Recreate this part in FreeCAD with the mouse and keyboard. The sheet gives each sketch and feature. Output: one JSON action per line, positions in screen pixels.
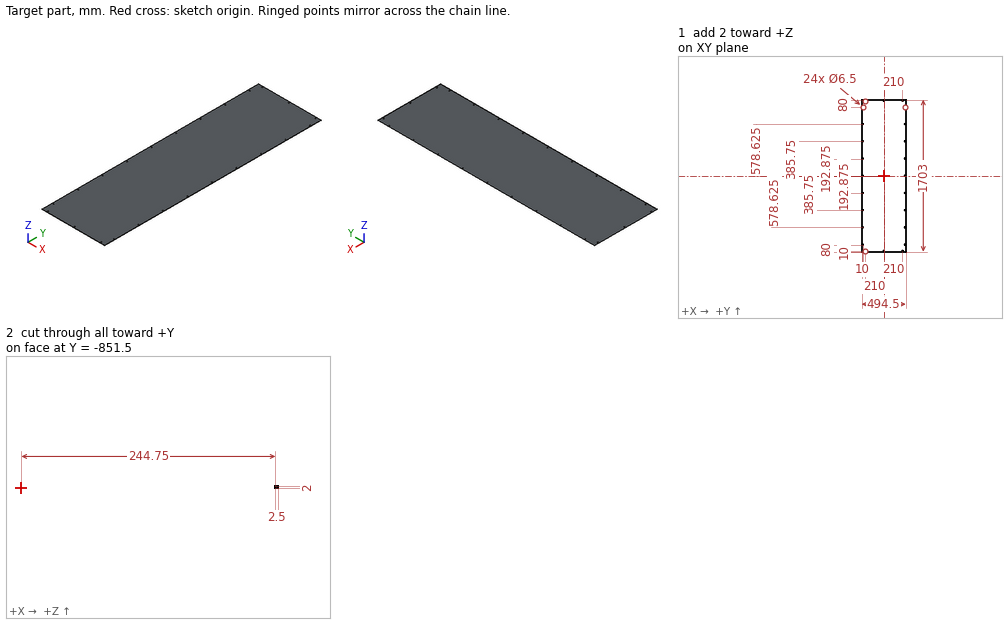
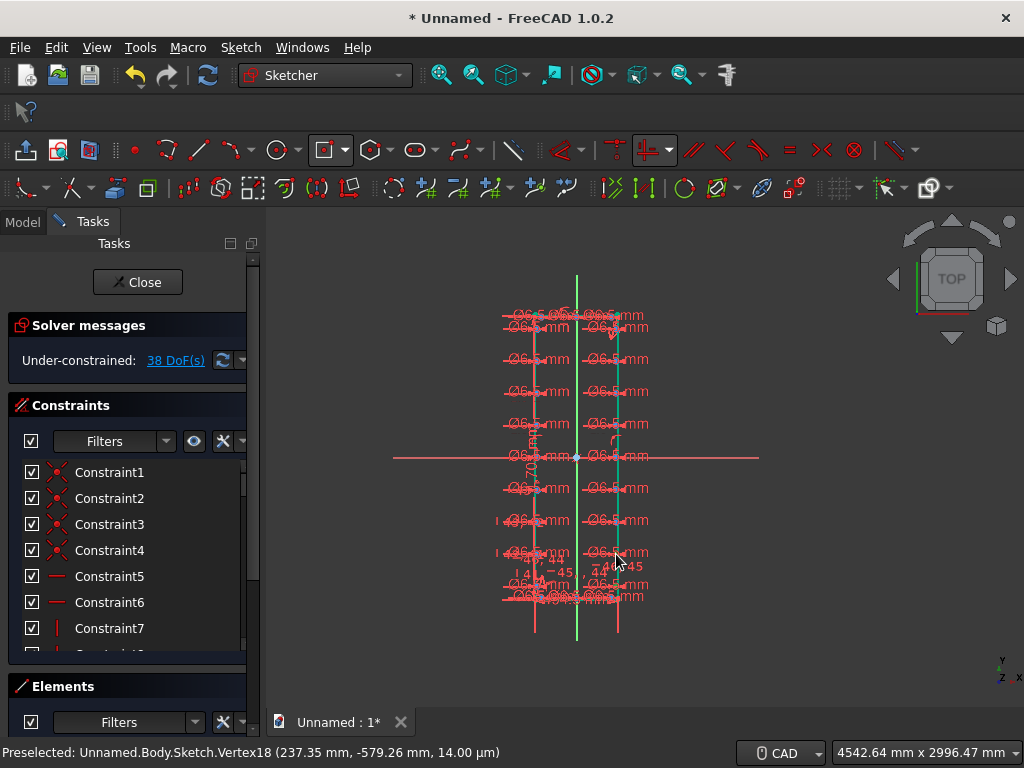
{"action": "key", "text": "v"}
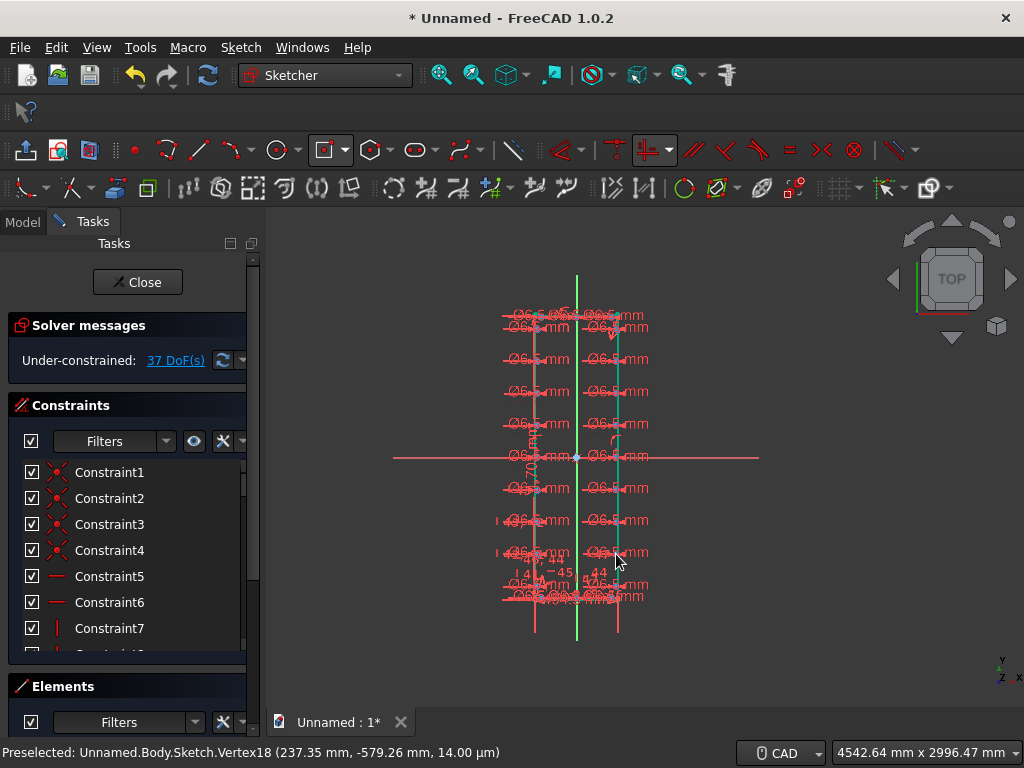
{"action": "left_click", "coordinate": [537, 554]}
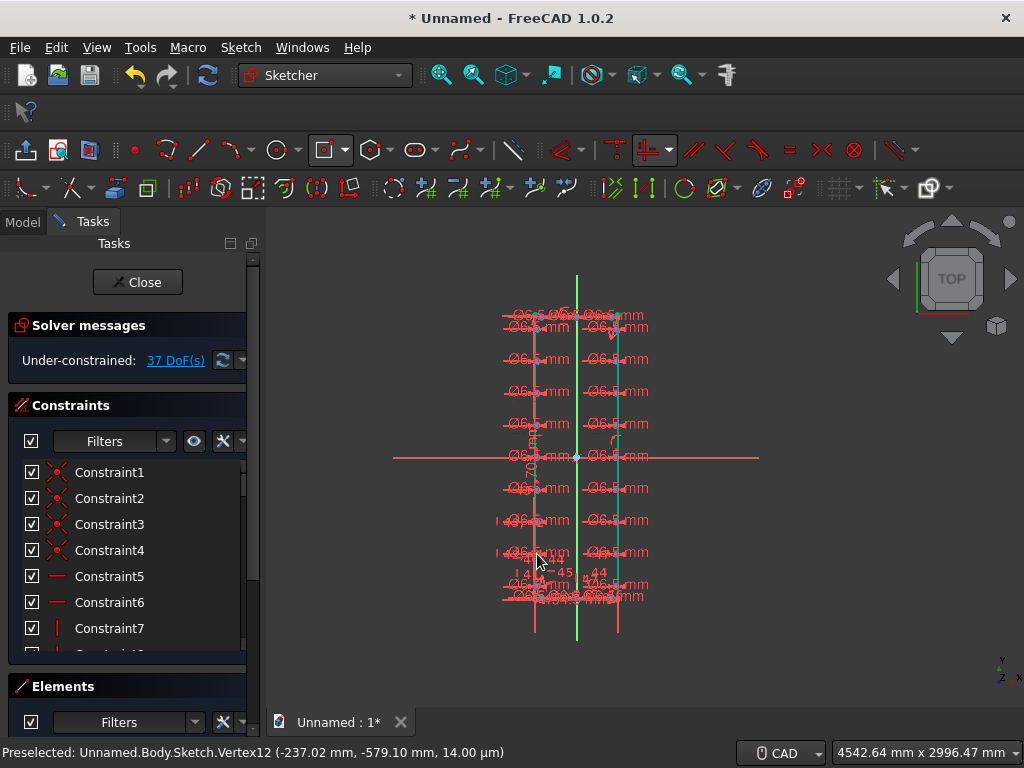
{"action": "left_click", "coordinate": [616, 554]}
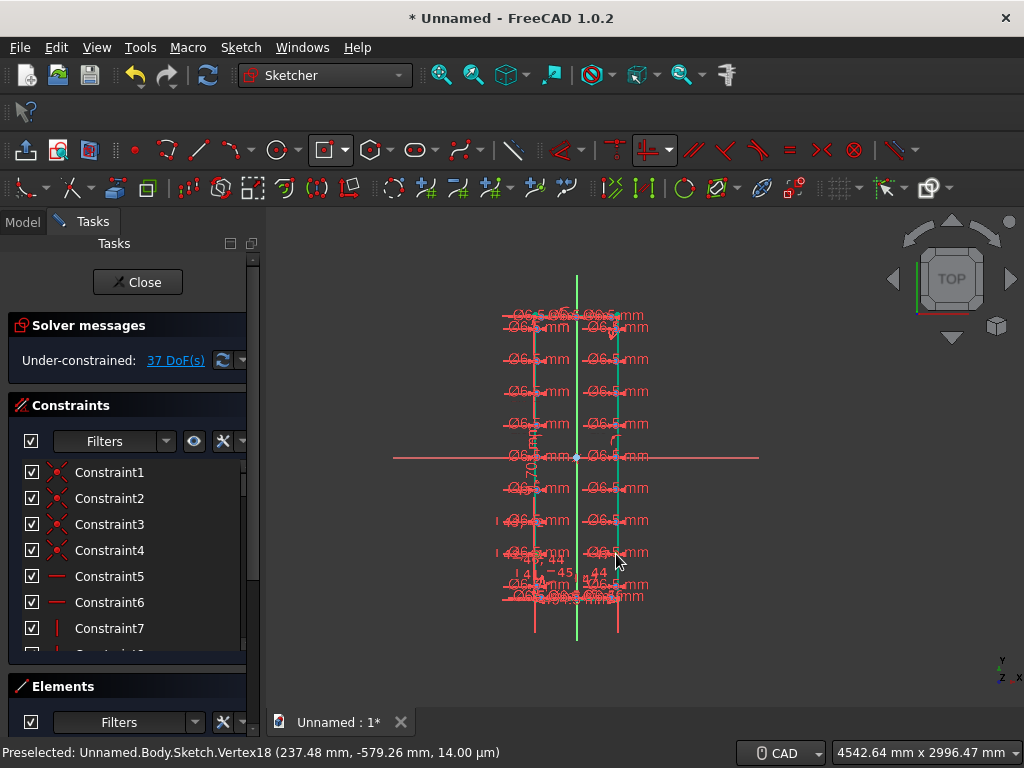
{"action": "key", "text": "h"}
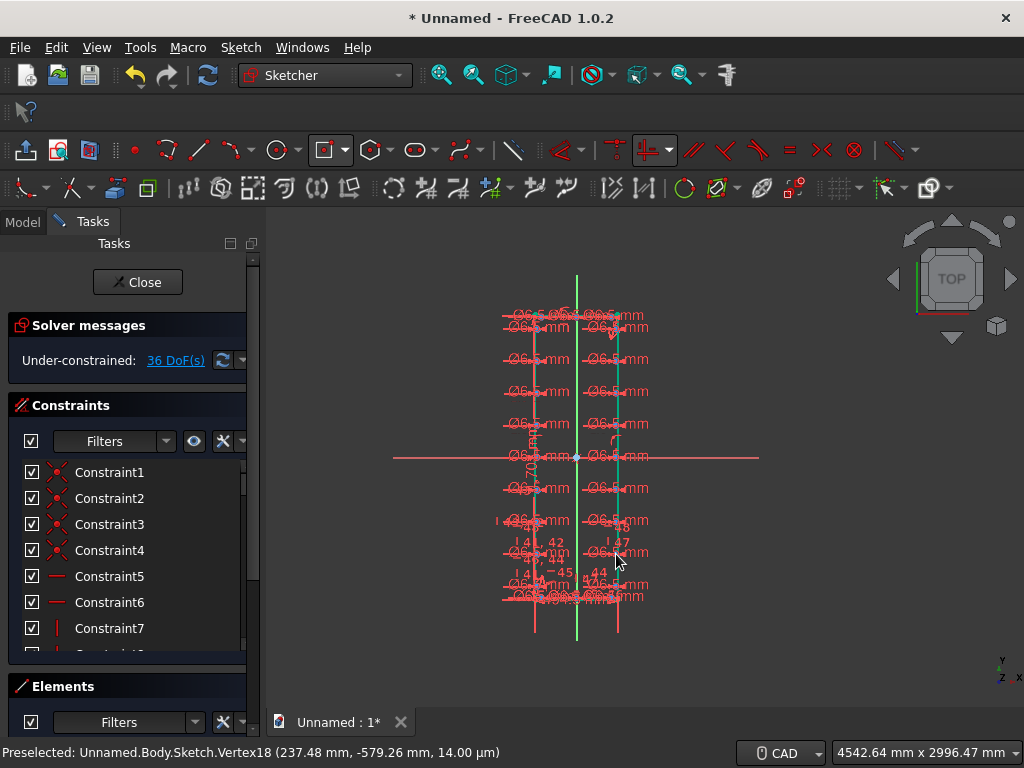
{"action": "left_click", "coordinate": [616, 554]}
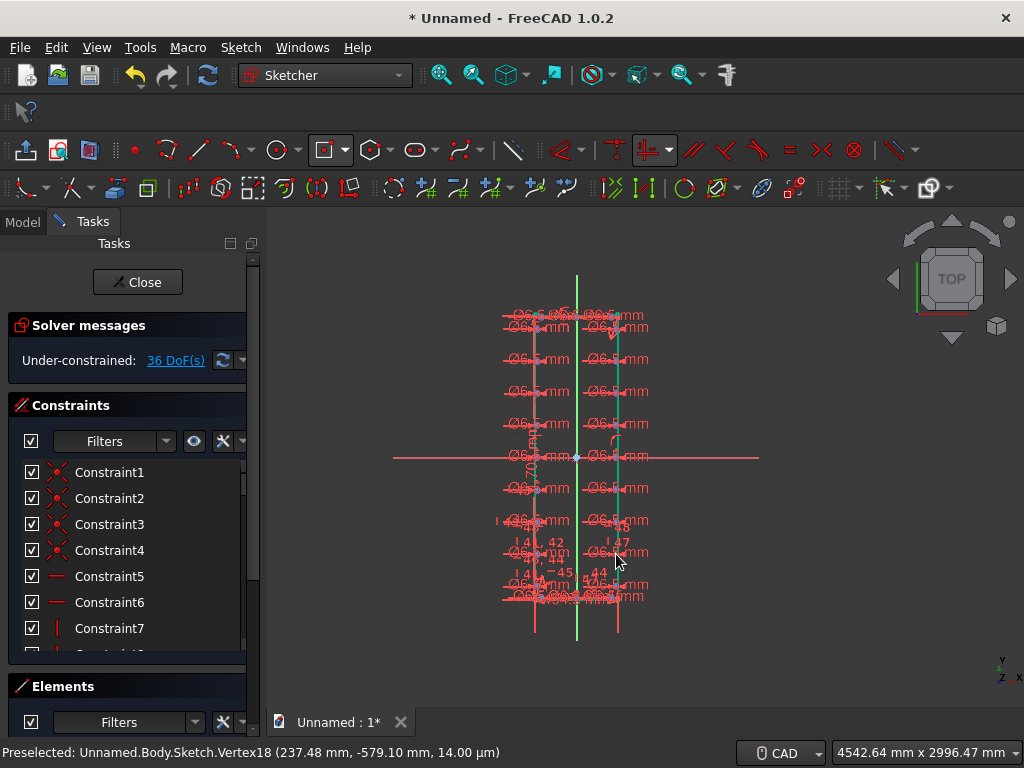
{"action": "scroll", "coordinate": [616, 522], "scroll_direction": "up", "scroll_amount": 4}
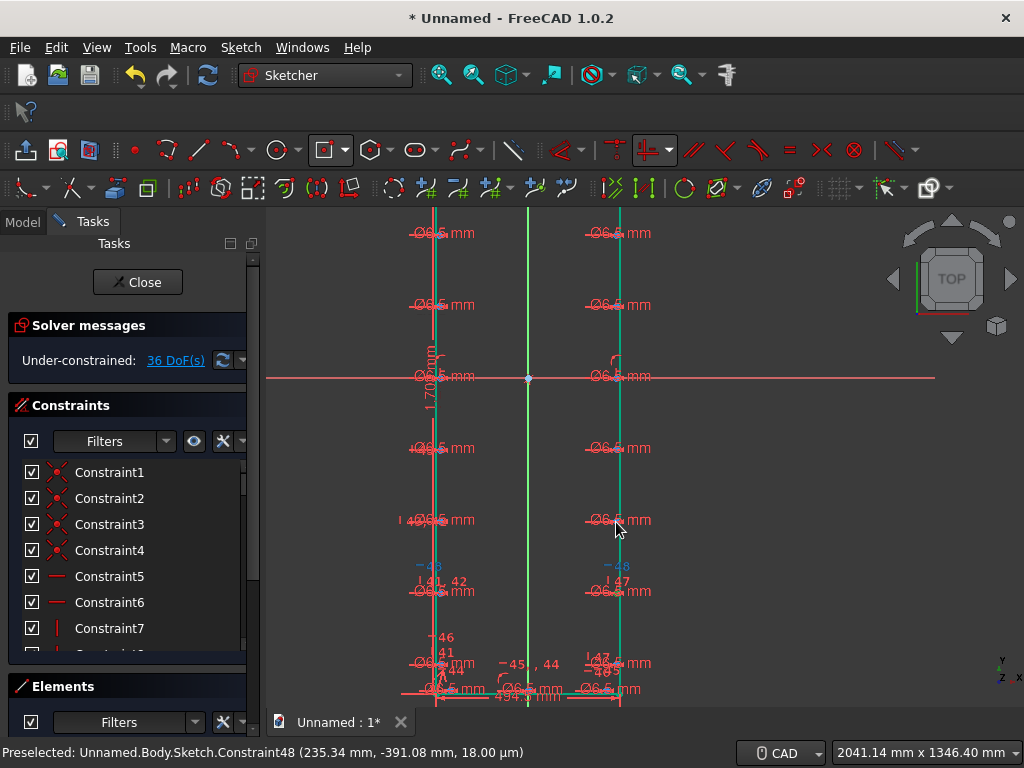
{"action": "left_click", "coordinate": [616, 522]}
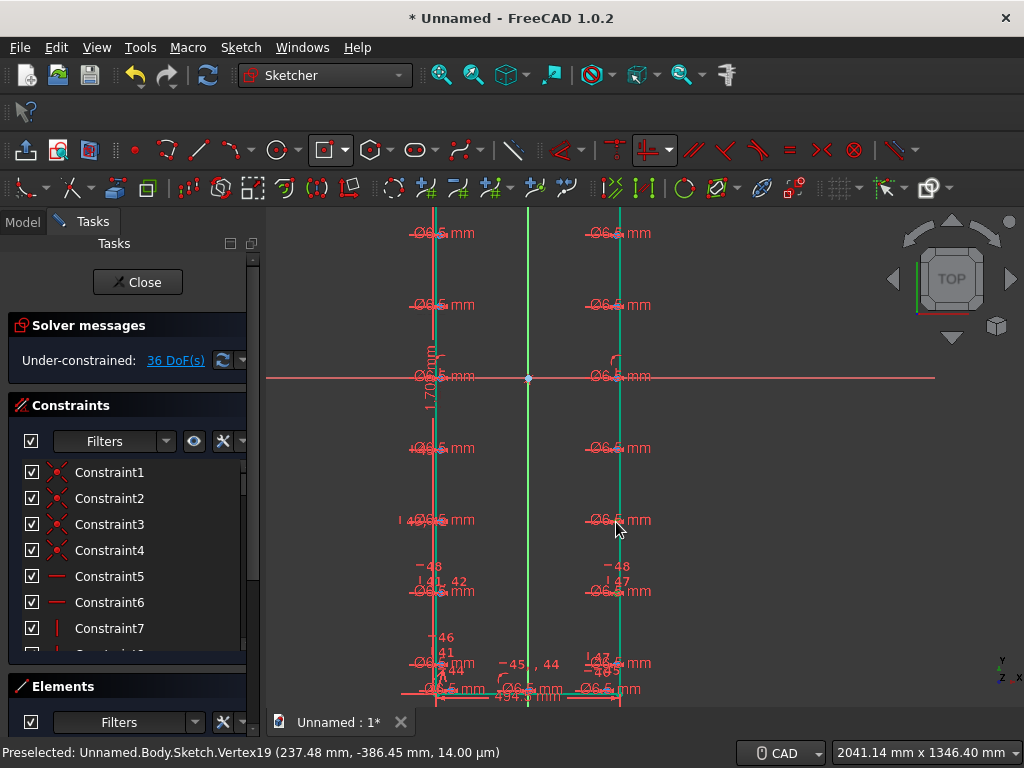
{"action": "key", "text": "v"}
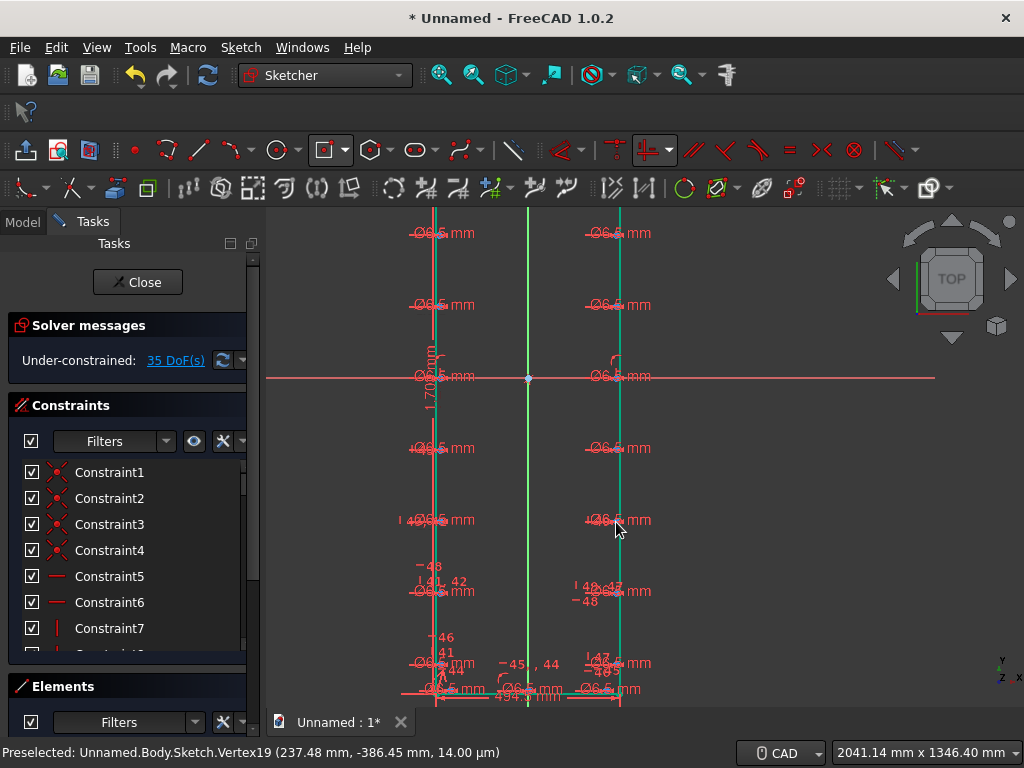
{"action": "left_click", "coordinate": [440, 522]}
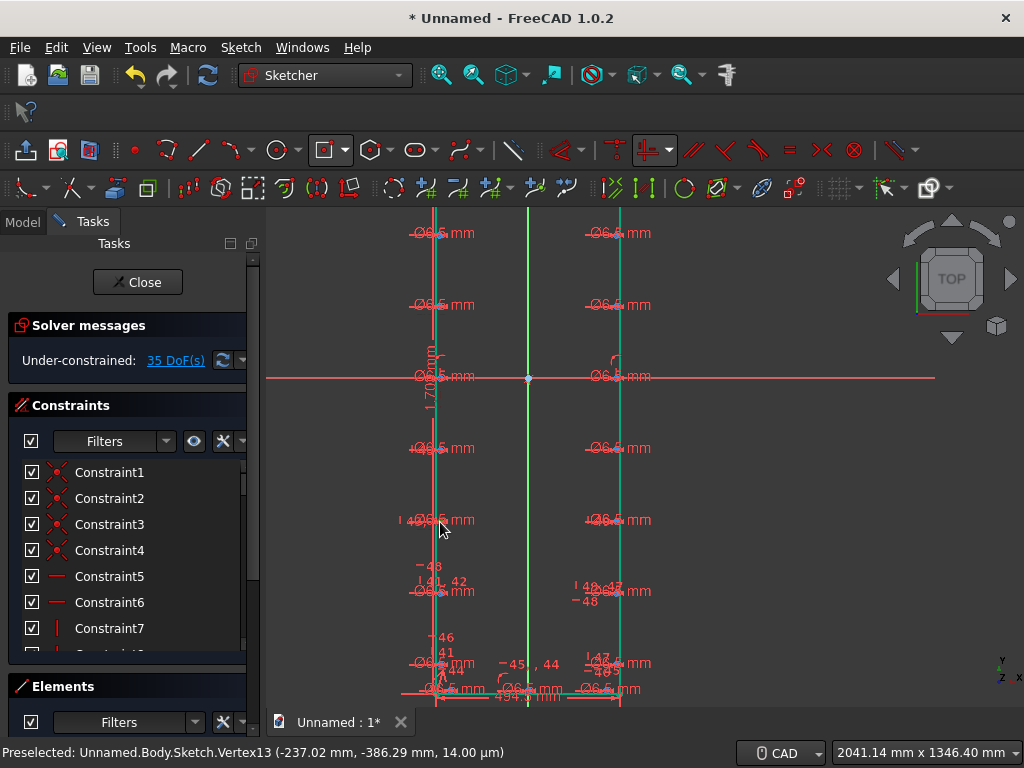
{"action": "left_click", "coordinate": [616, 522]}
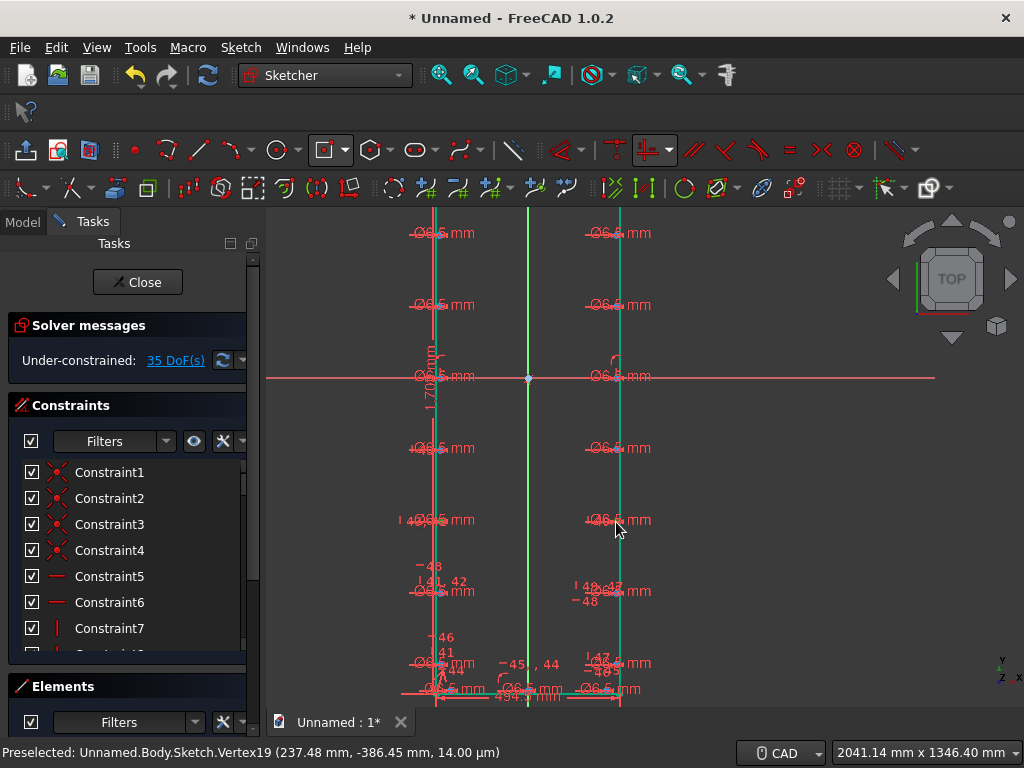
{"action": "key", "text": "h"}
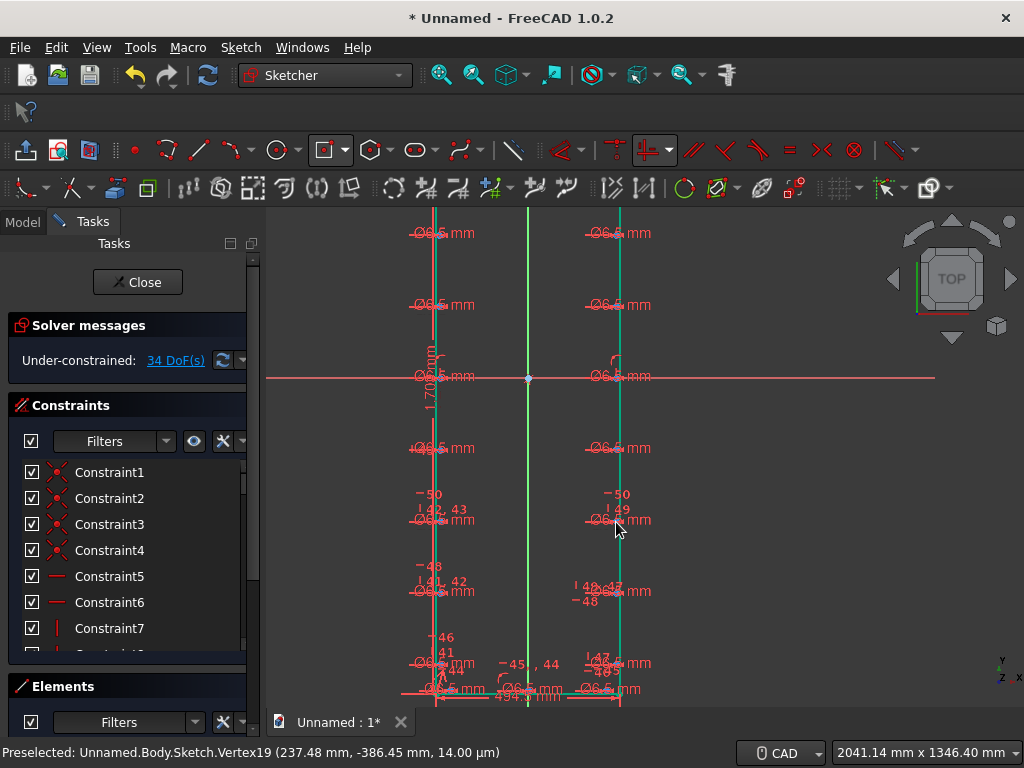
{"action": "left_click", "coordinate": [616, 522]}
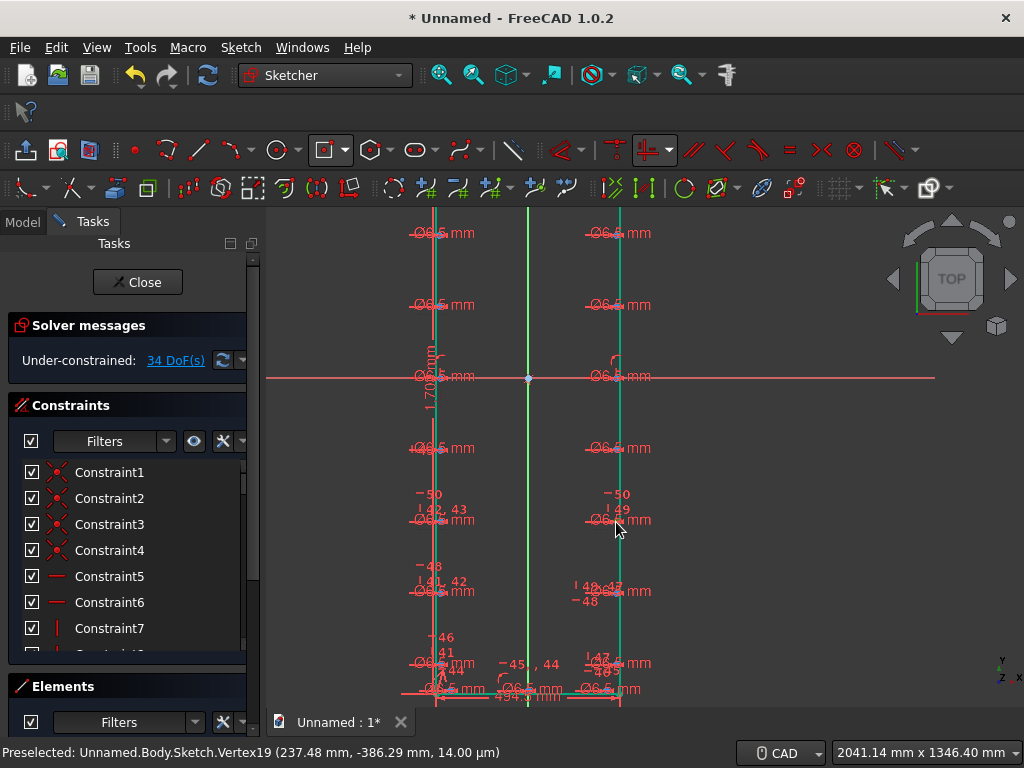
{"action": "left_click", "coordinate": [616, 450]}